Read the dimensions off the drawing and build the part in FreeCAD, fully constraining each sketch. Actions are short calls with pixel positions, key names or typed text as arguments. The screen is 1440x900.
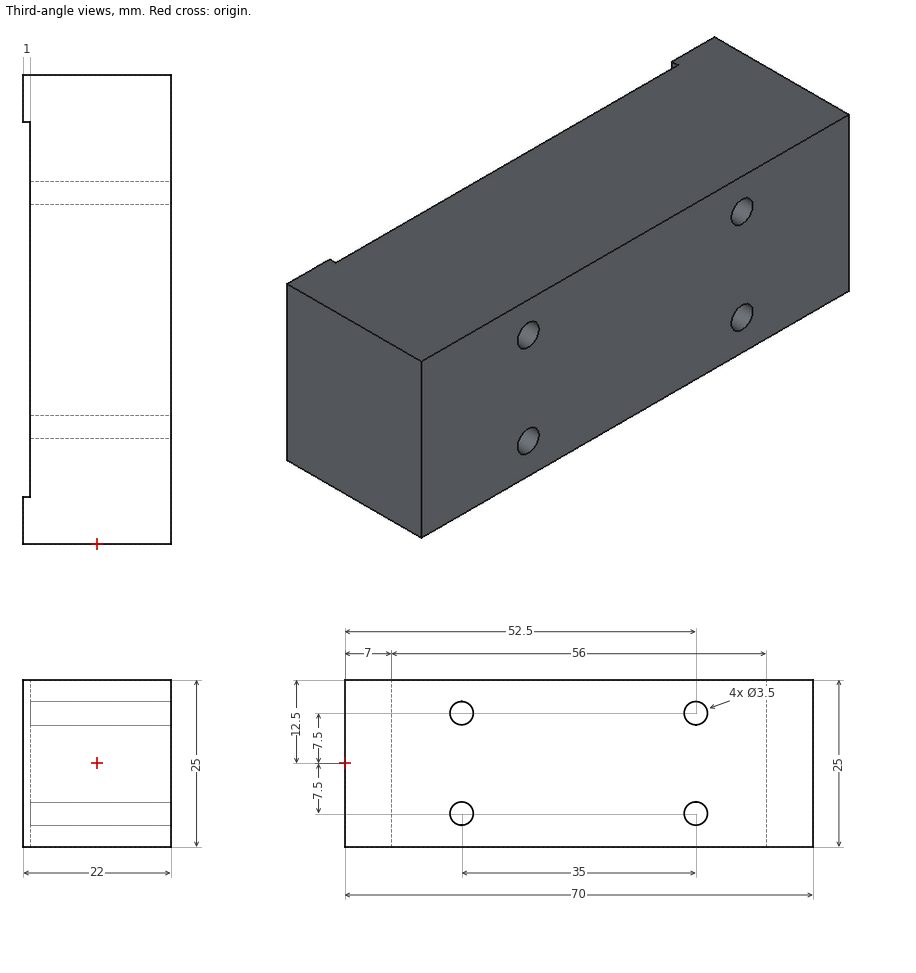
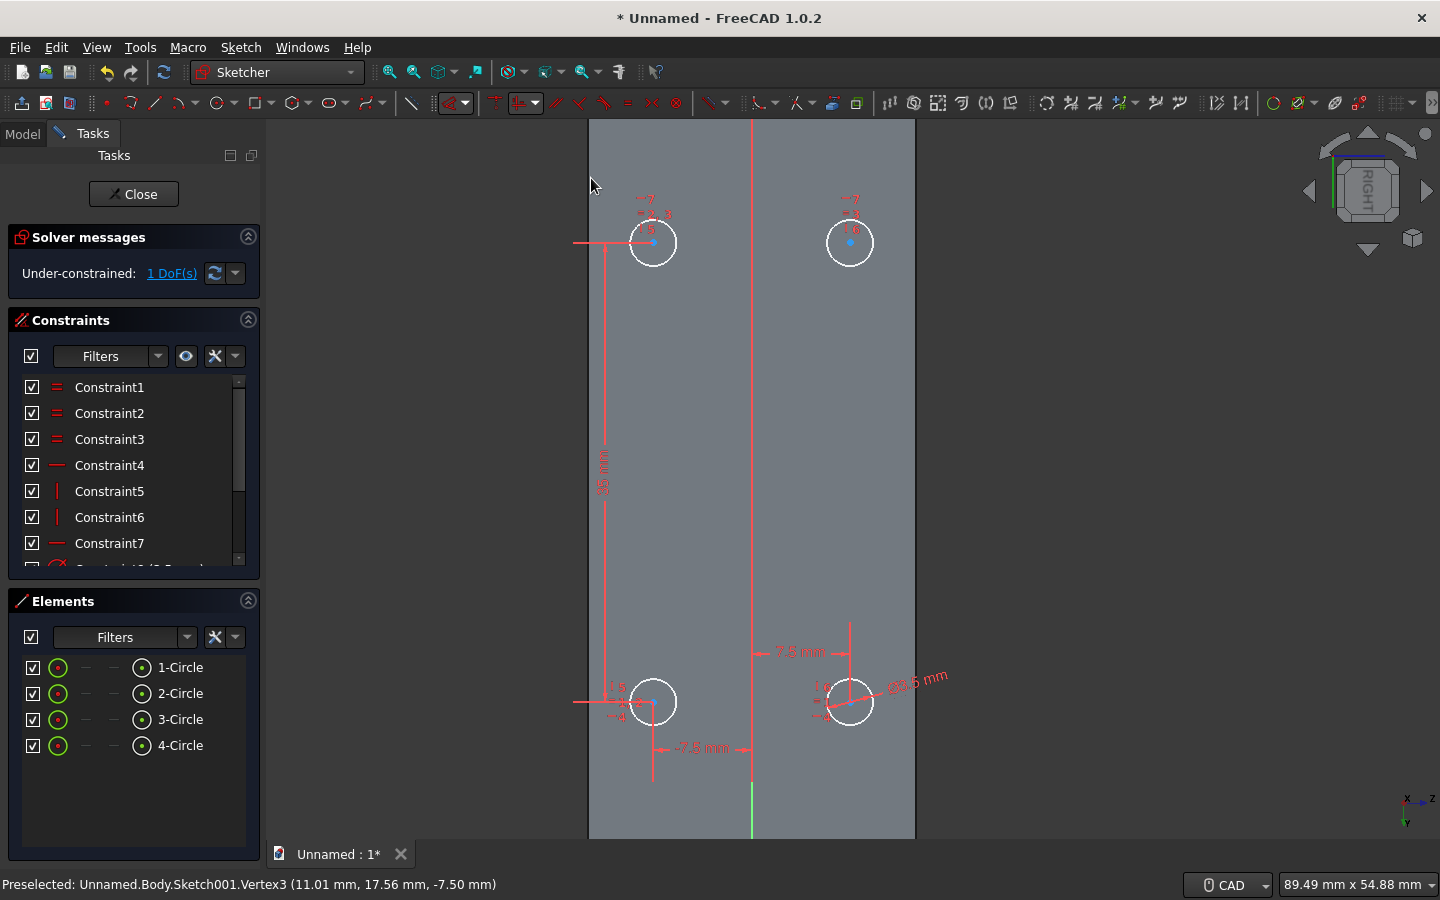
click(850, 702)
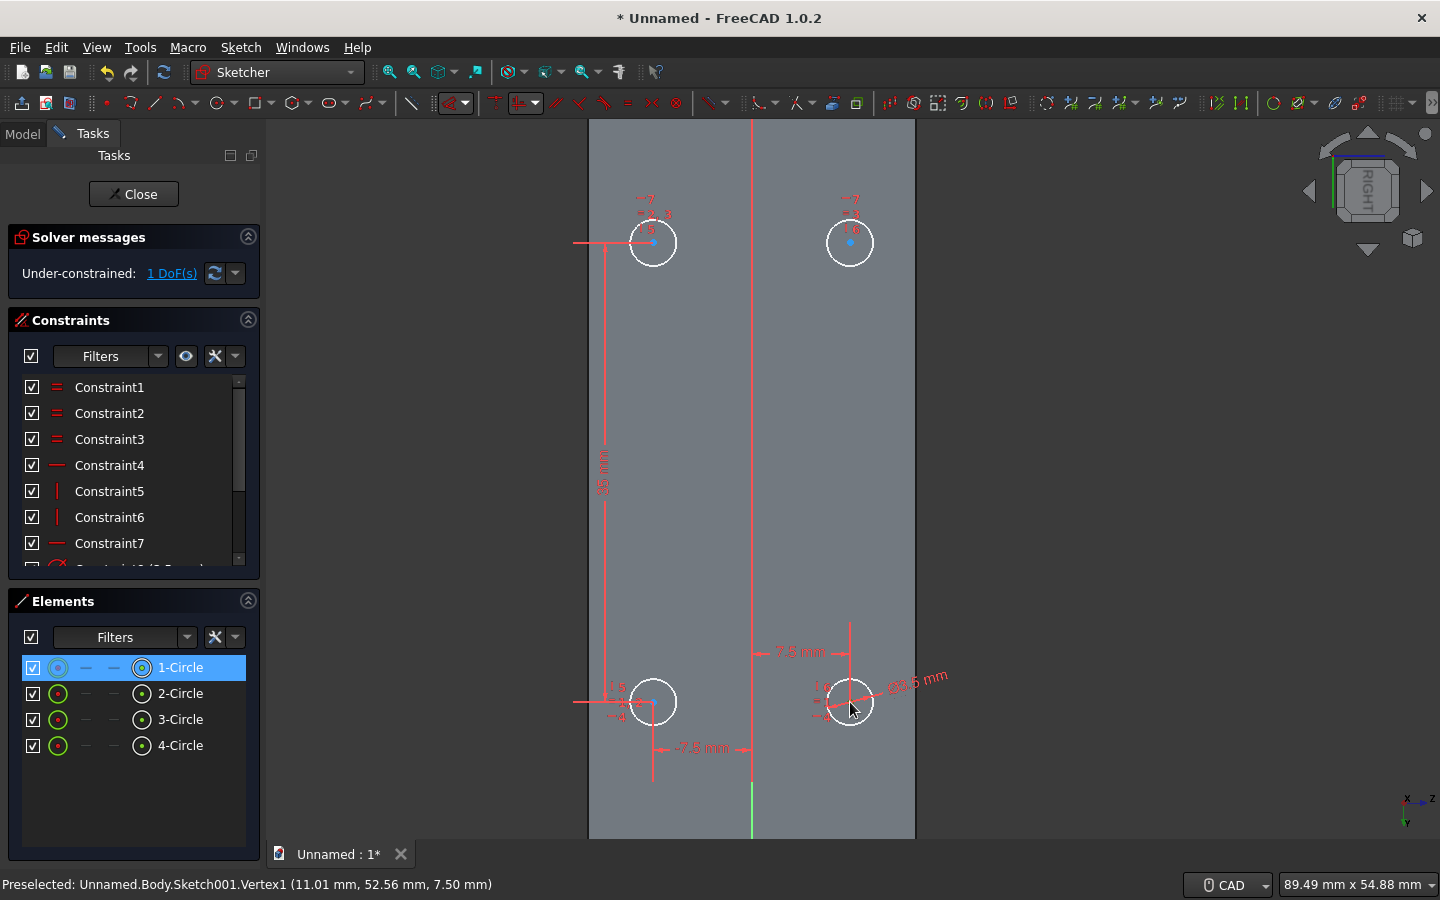
click(468, 104)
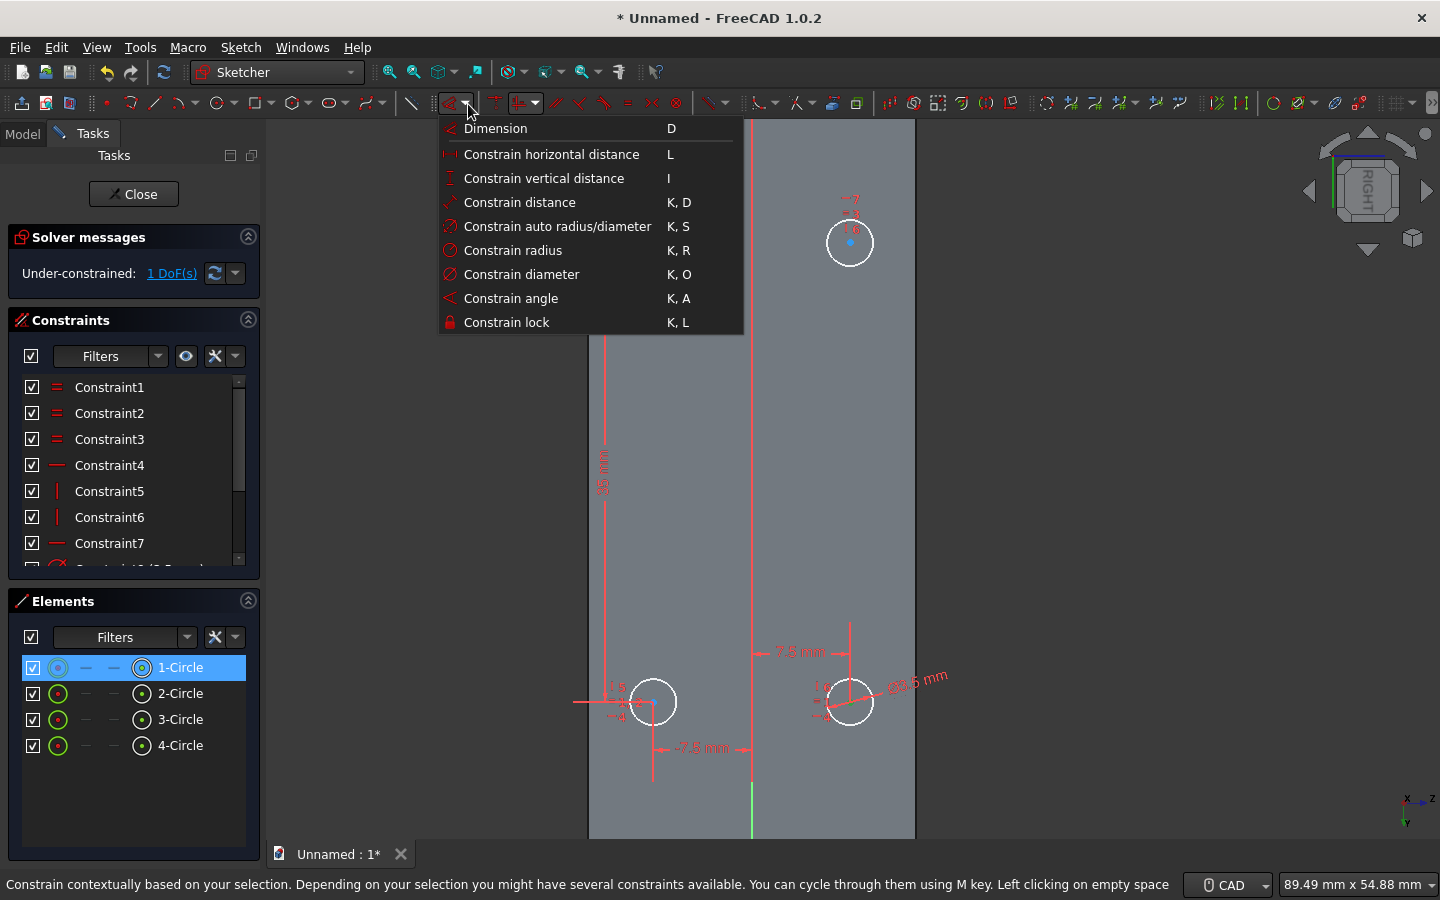
click(591, 178)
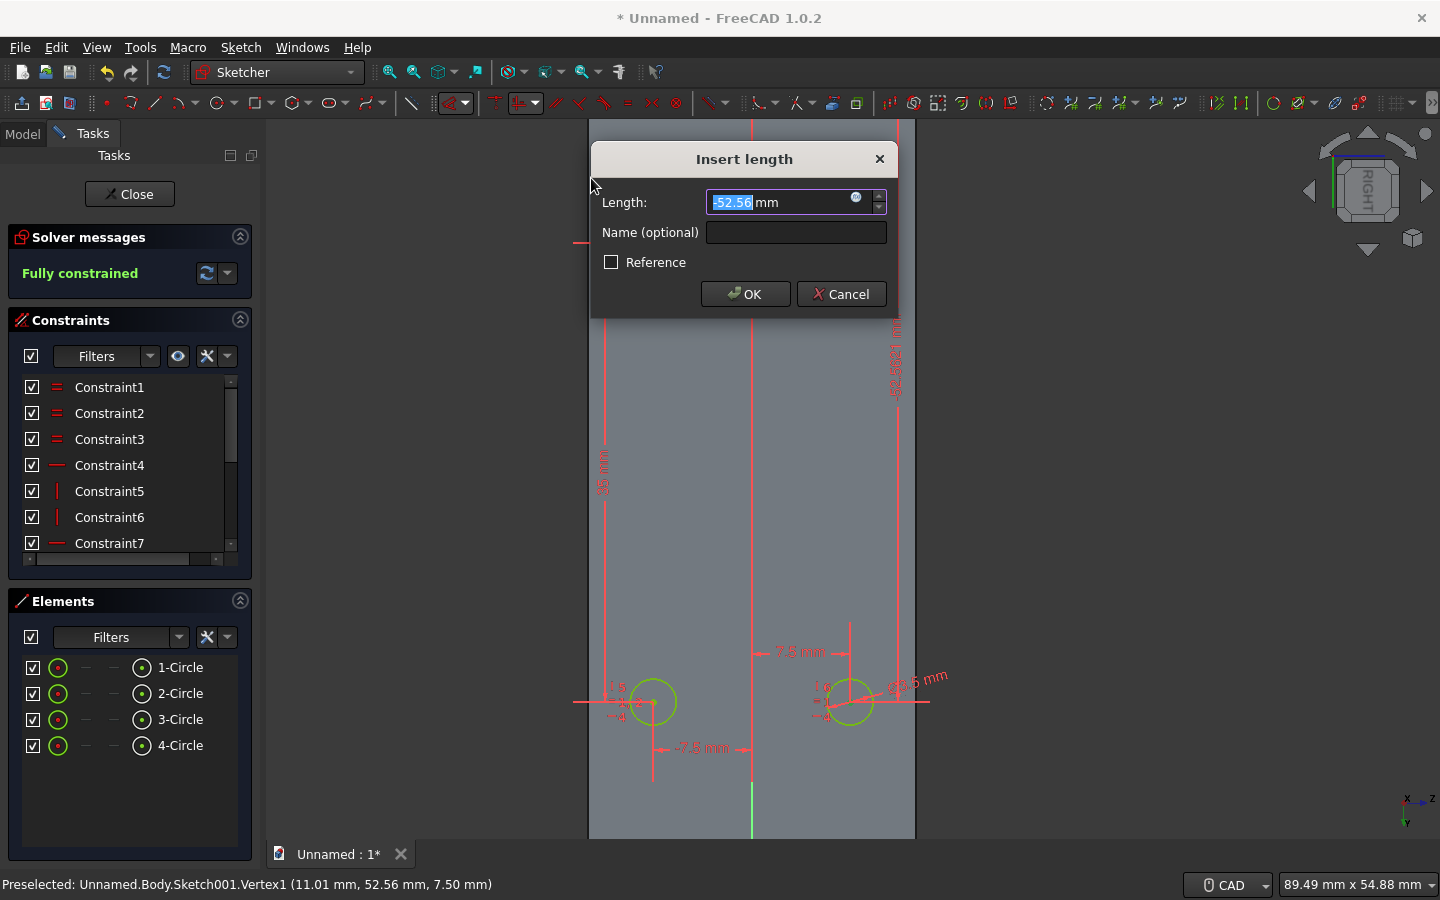
text(-52.5)
key(Return)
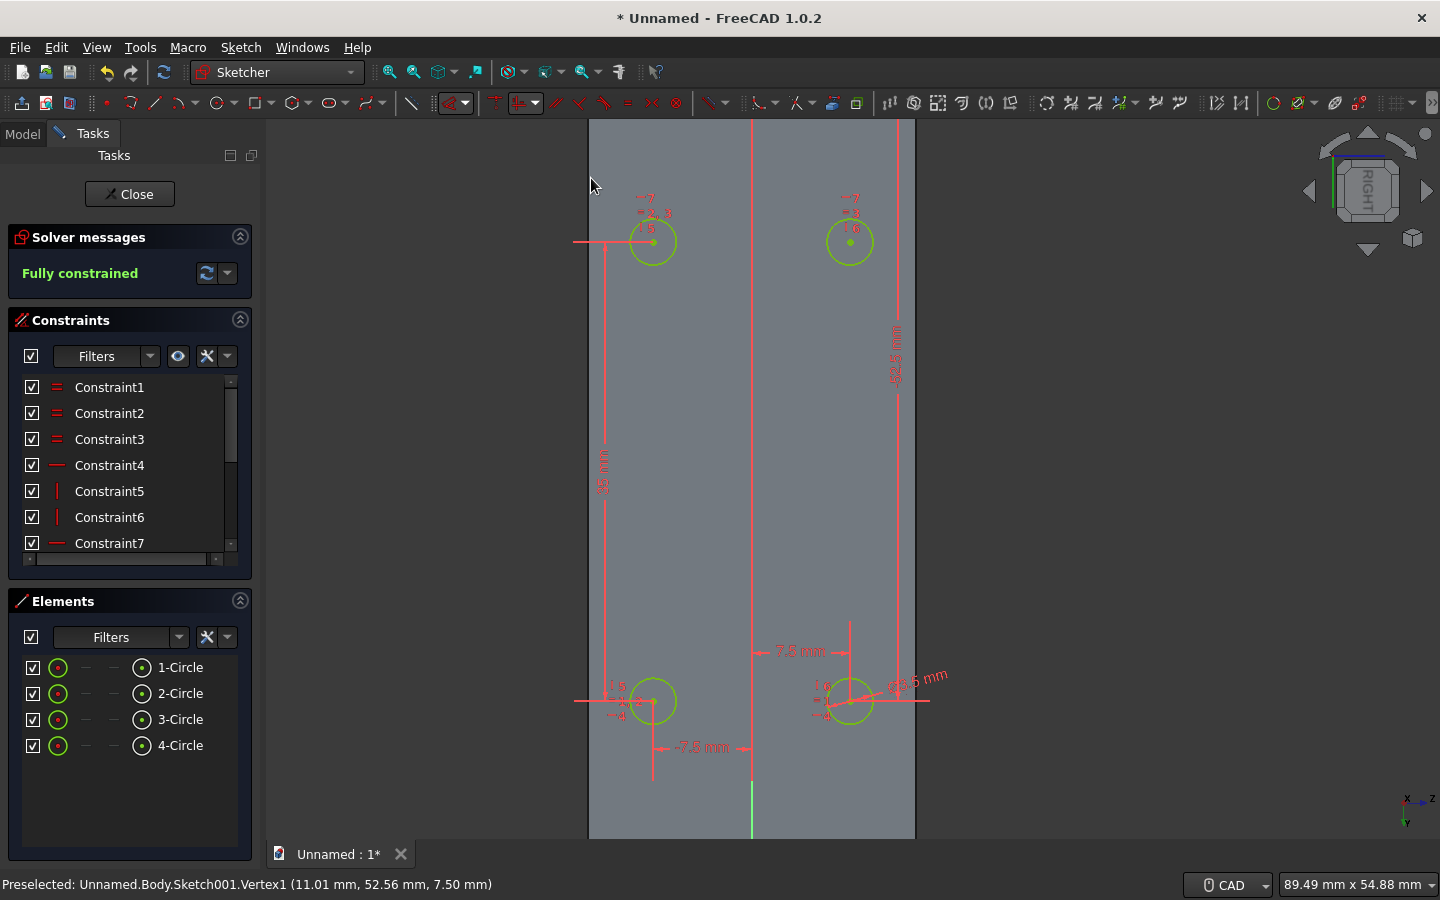
click(130, 194)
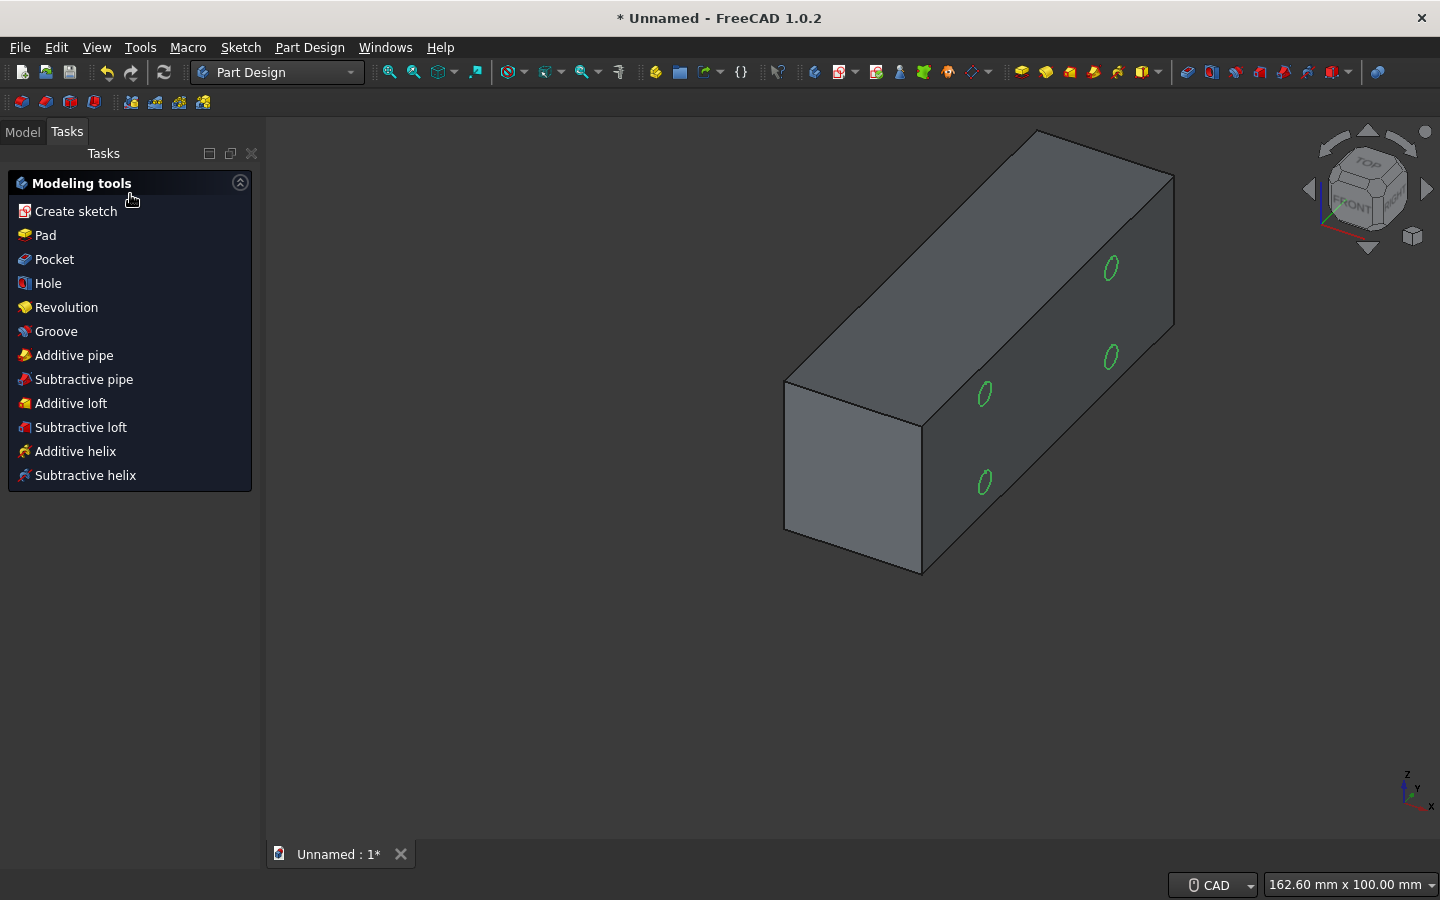
click(1188, 72)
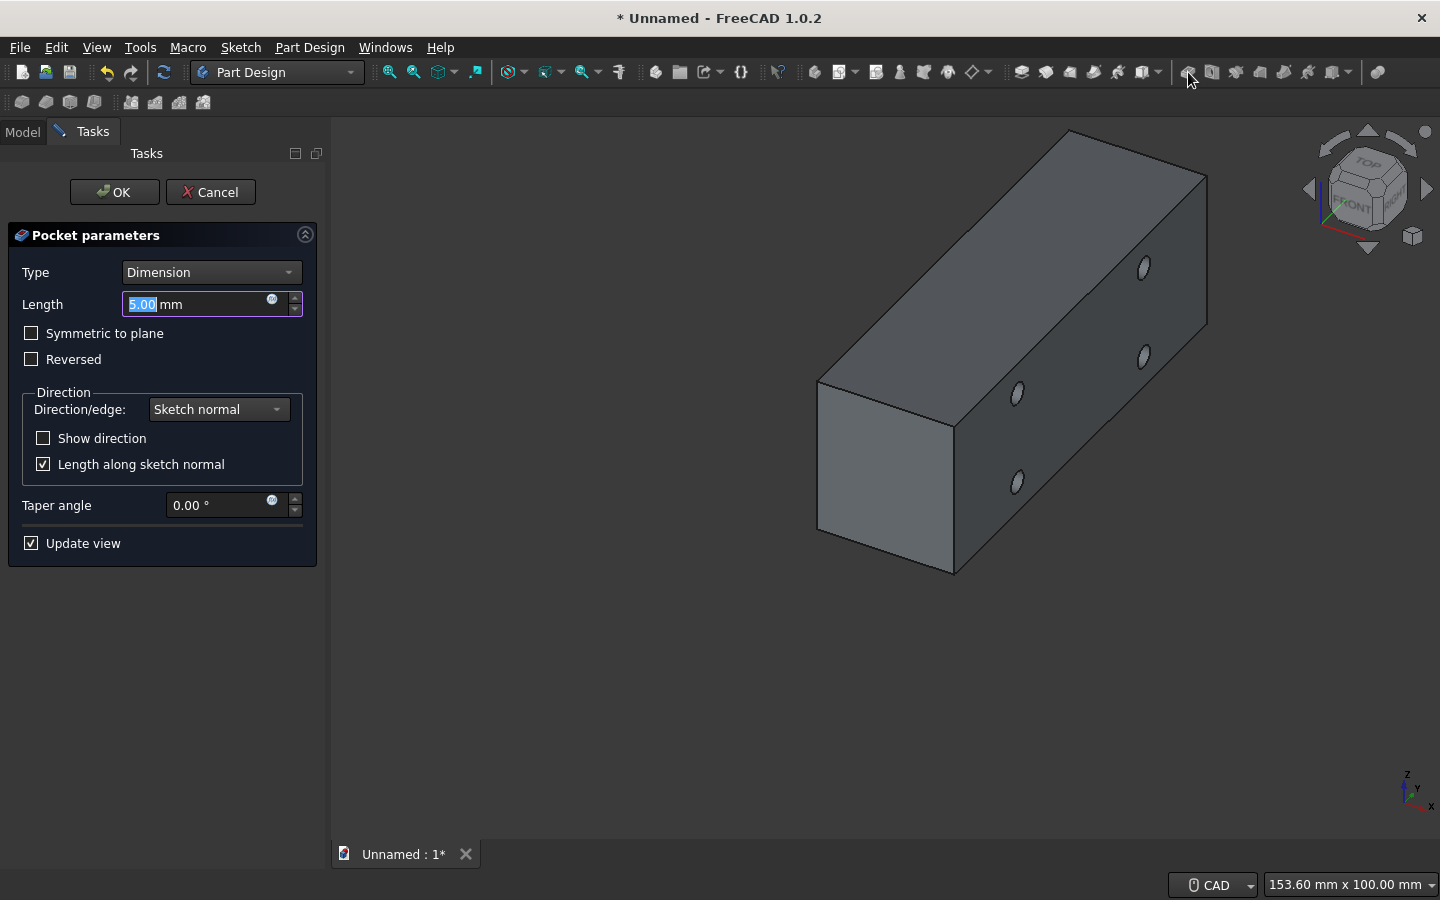
click(212, 272)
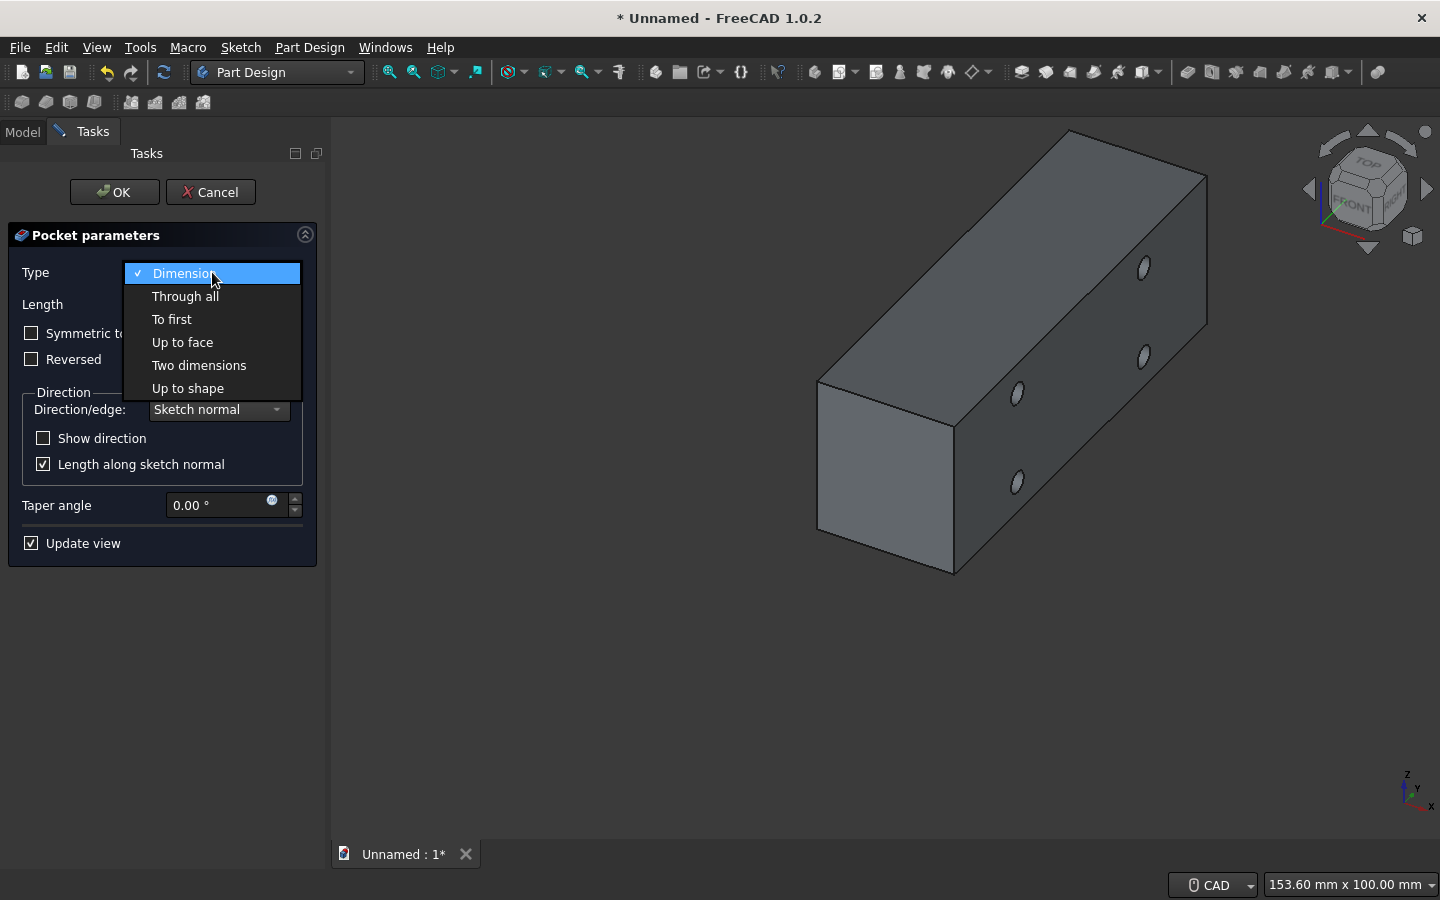
click(212, 296)